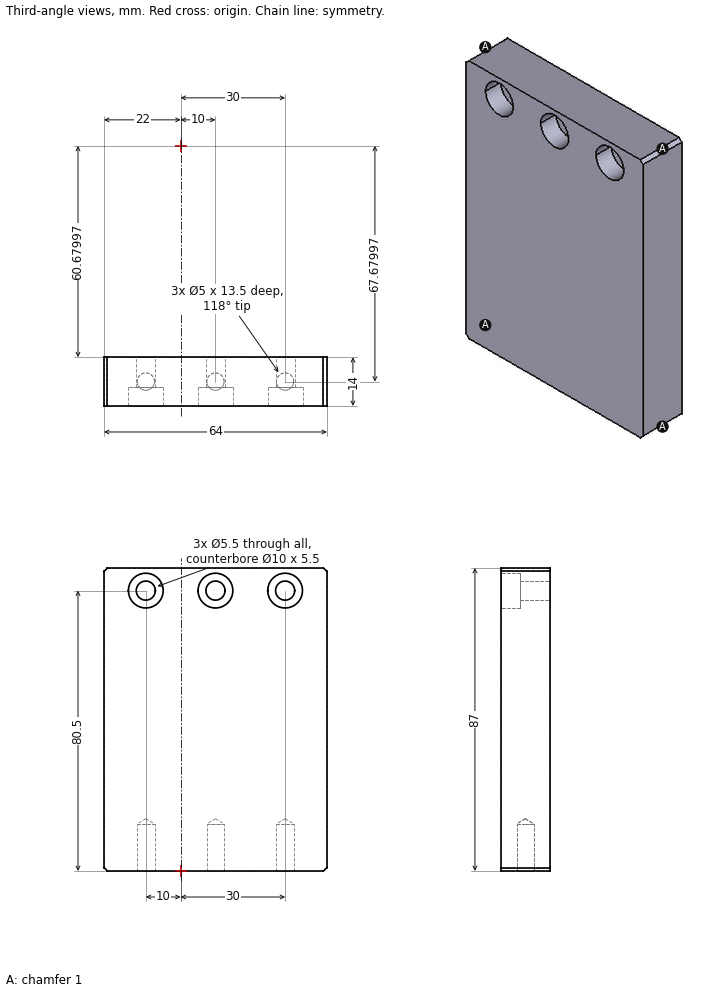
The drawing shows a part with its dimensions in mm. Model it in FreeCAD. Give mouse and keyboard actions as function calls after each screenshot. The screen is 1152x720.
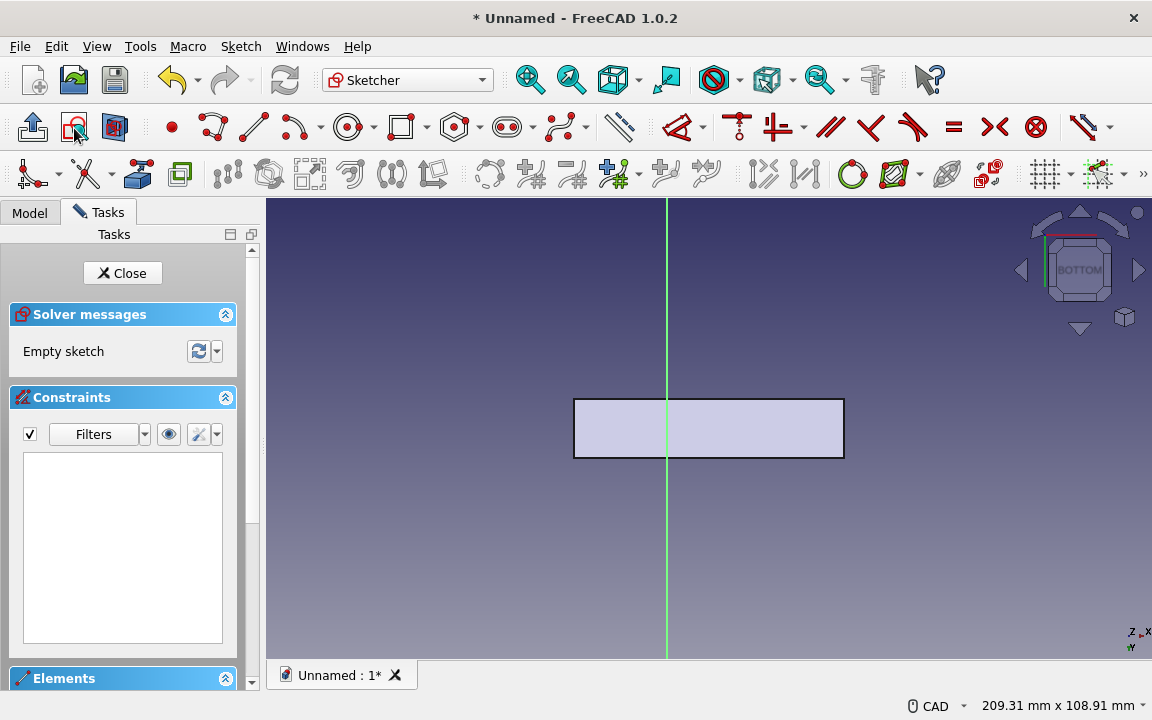
scroll(501, 226, down, 2)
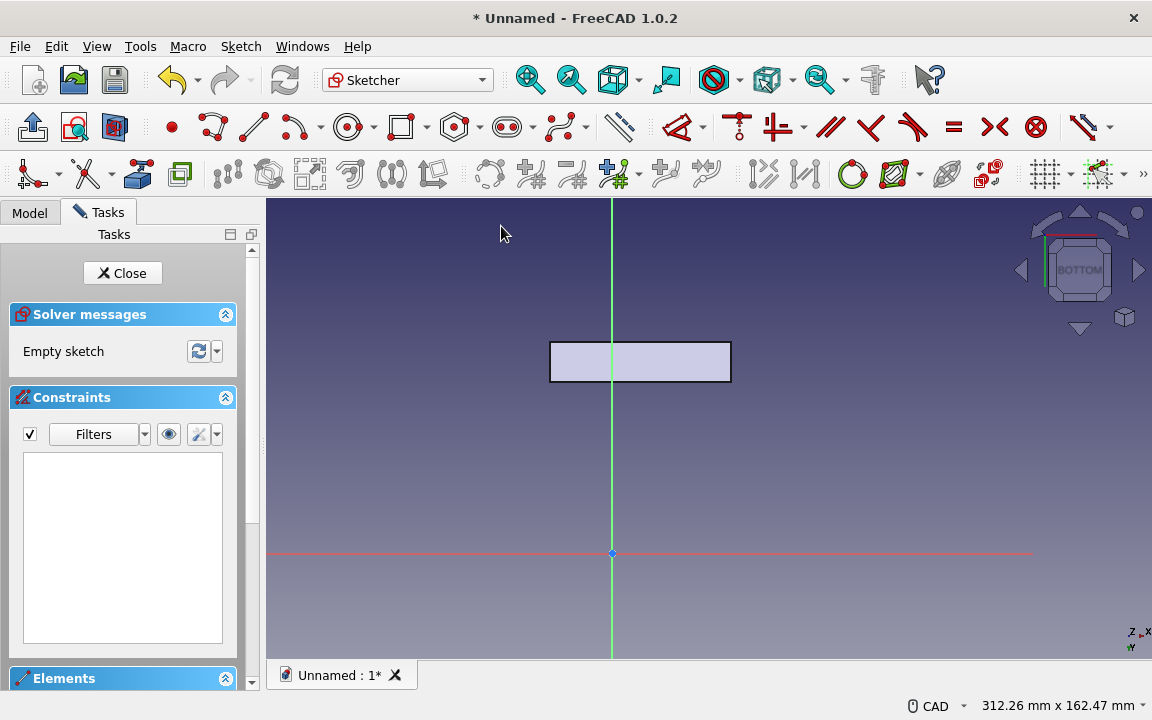
scroll(641, 507, up, 2)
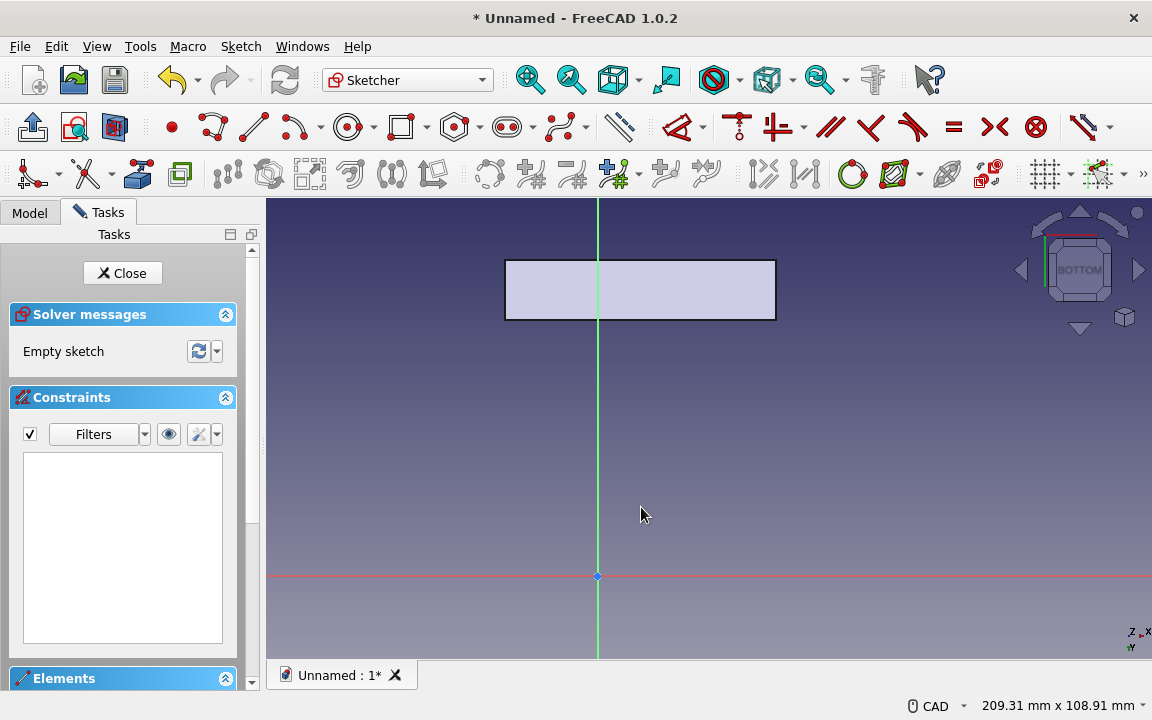
click(348, 128)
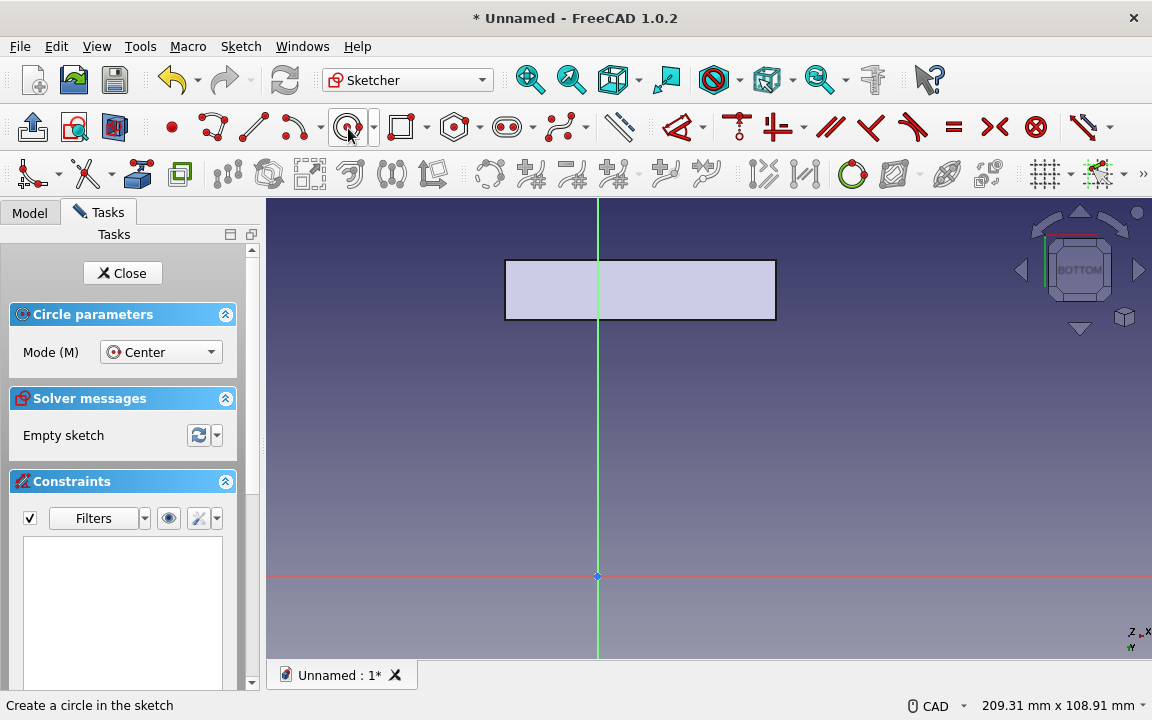
scroll(725, 290, up, 4)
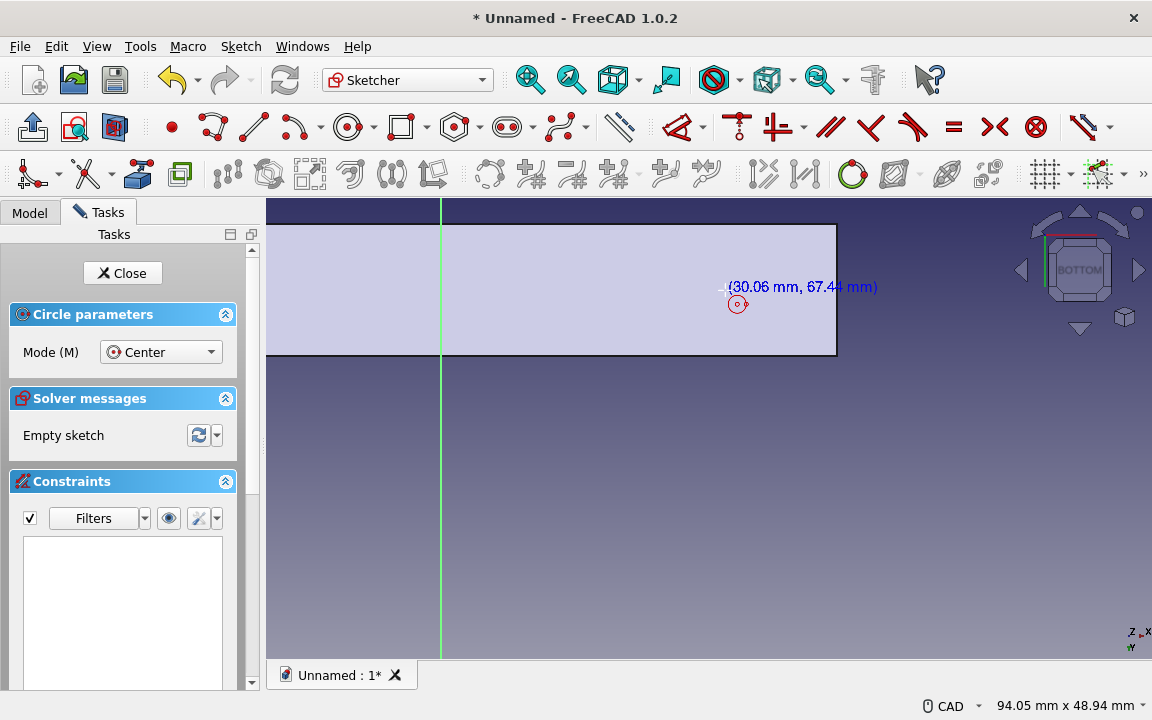
click(724, 290)
move(740, 273)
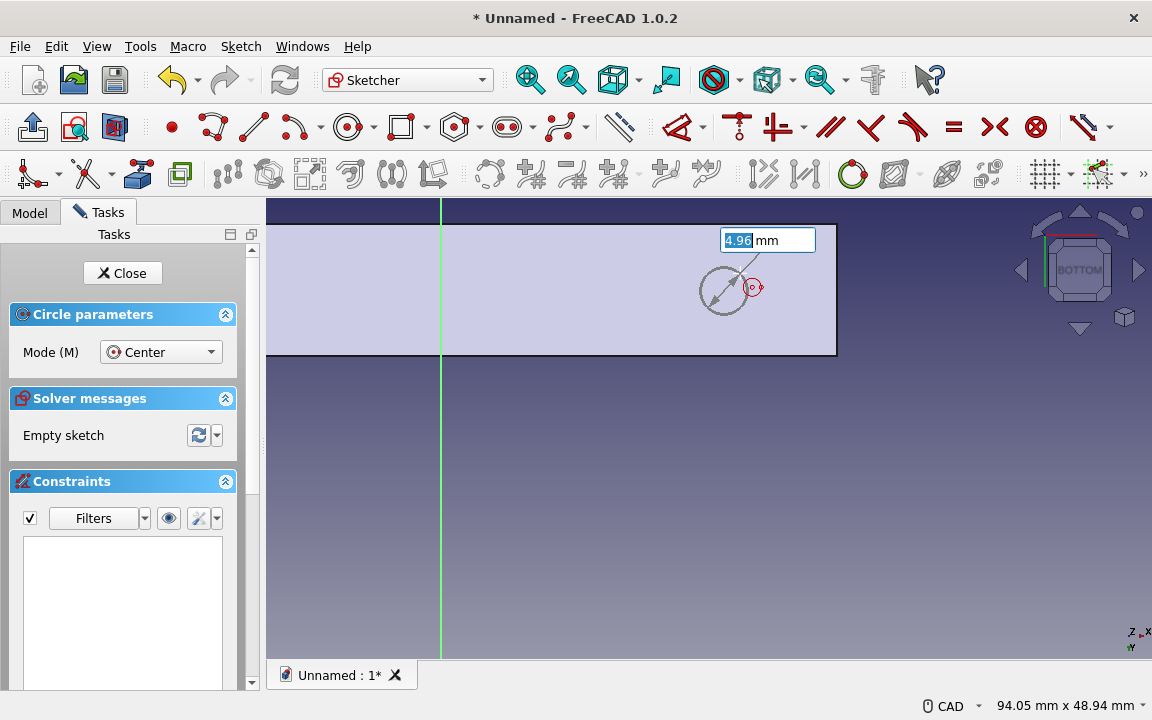
text(5)
key(Return)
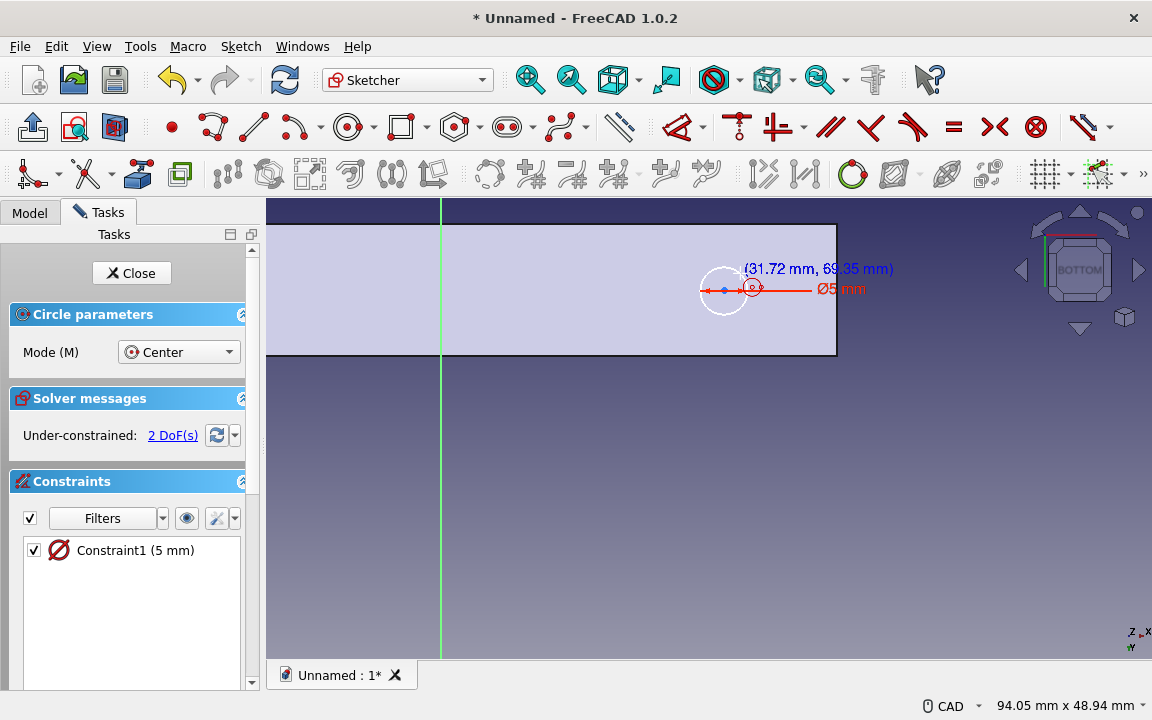
click(535, 290)
move(552, 273)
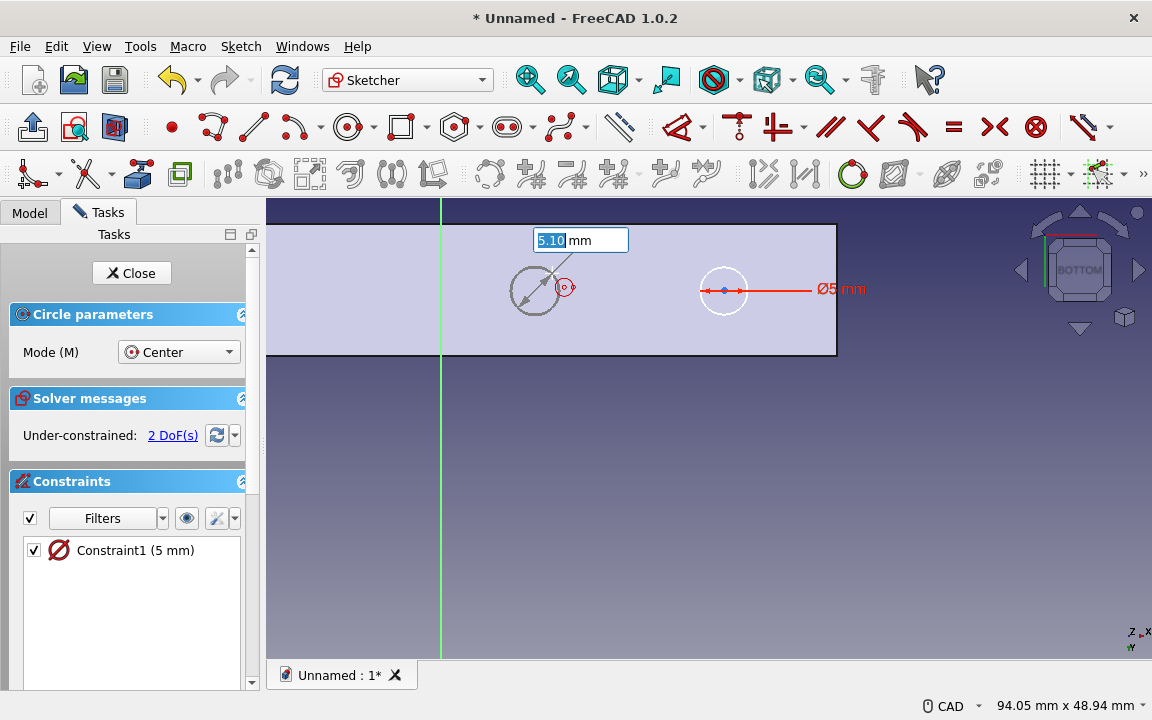
text(5)
key(Return)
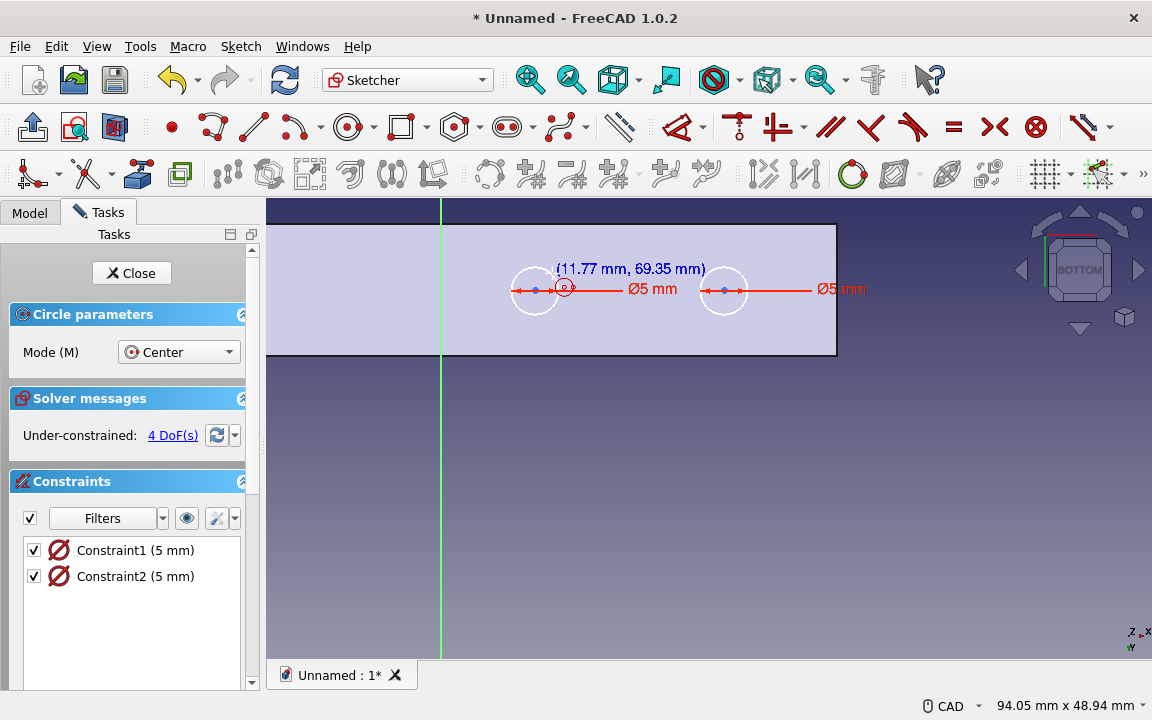
click(347, 290)
move(364, 273)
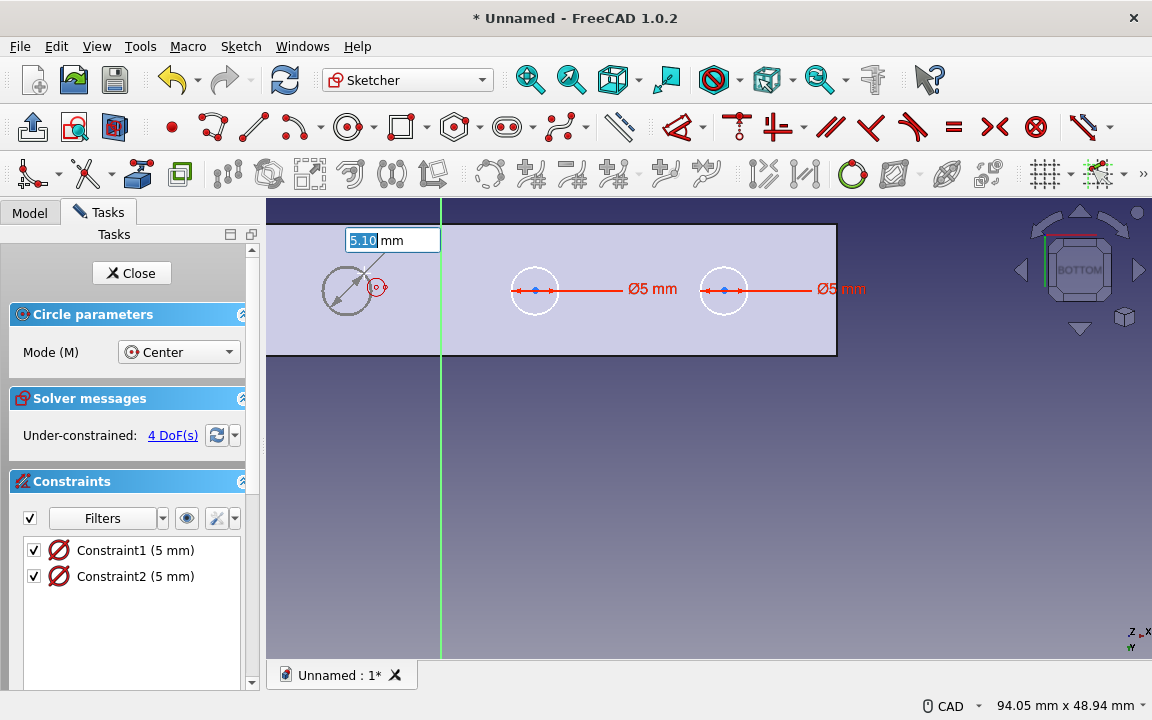
text(5)
key(Return)
key(Escape)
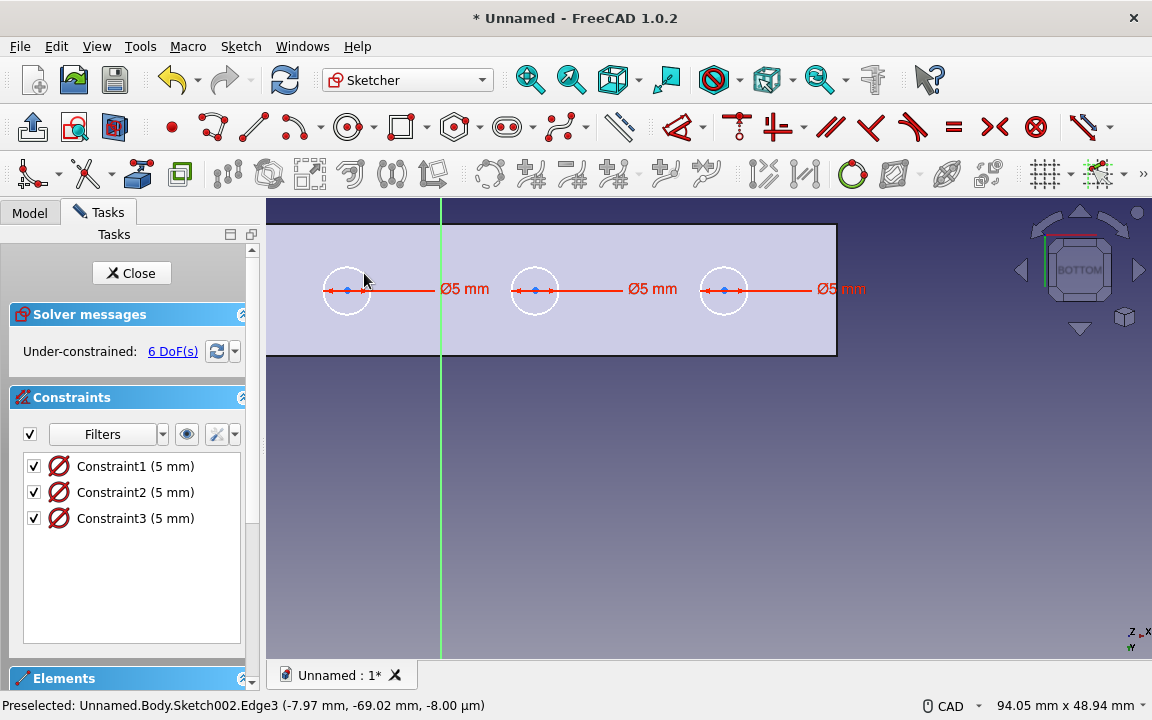
click(535, 291)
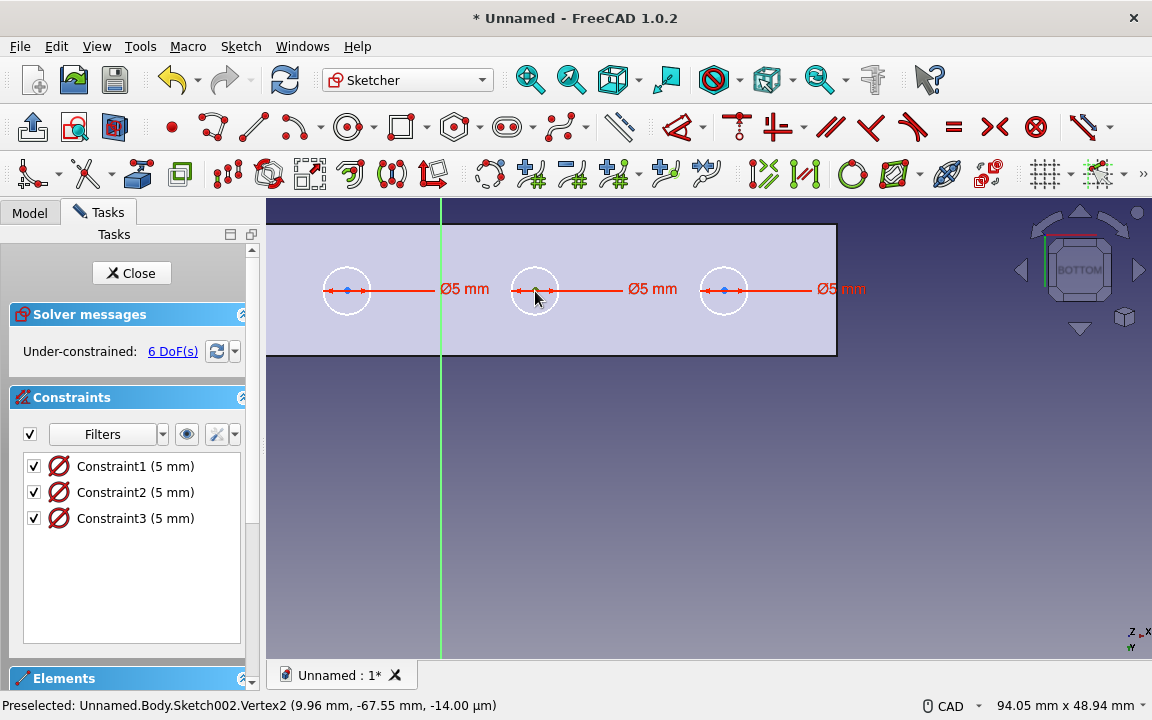
click(347, 291)